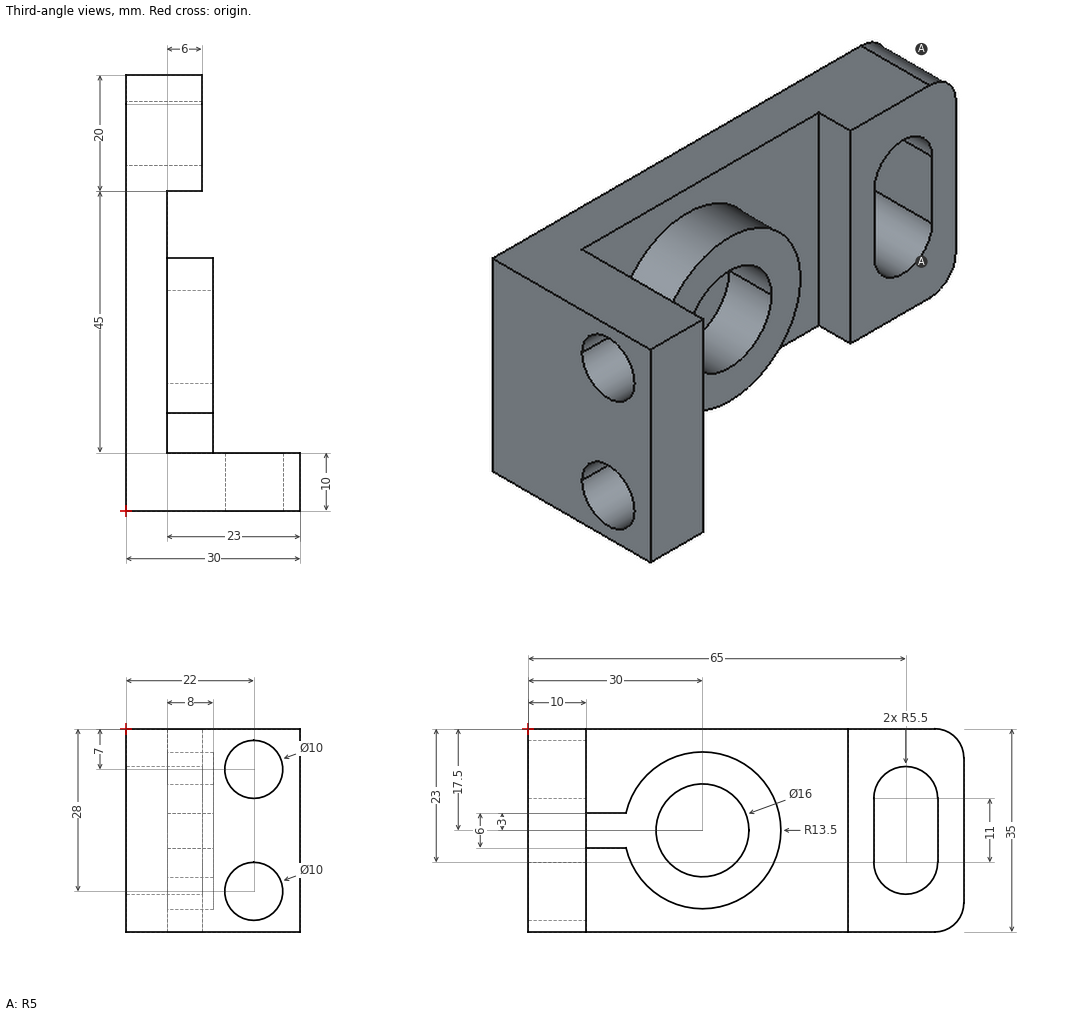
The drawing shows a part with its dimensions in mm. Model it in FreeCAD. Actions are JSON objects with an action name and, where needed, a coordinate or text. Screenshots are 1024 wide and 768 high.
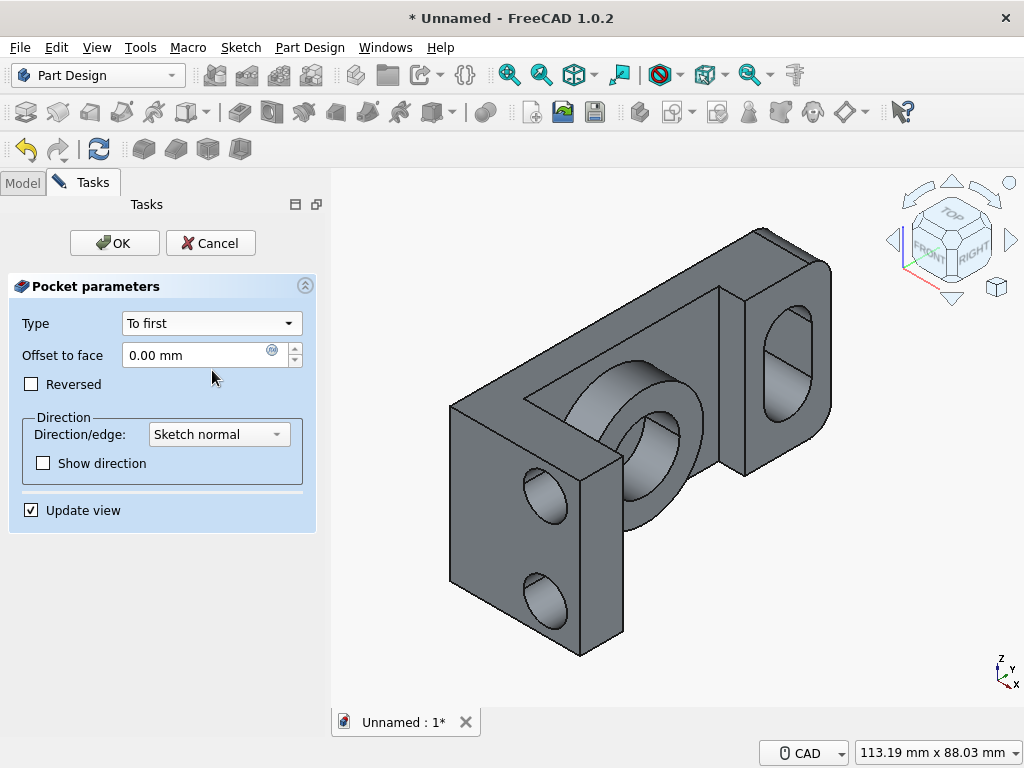
{"action": "left_click", "coordinate": [115, 243]}